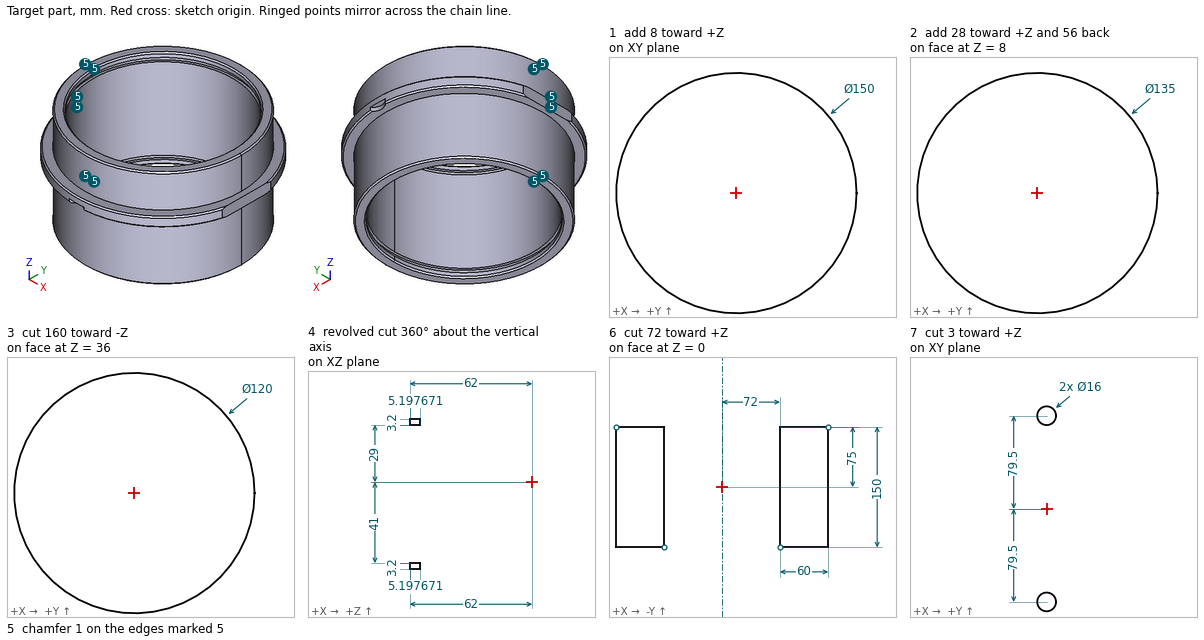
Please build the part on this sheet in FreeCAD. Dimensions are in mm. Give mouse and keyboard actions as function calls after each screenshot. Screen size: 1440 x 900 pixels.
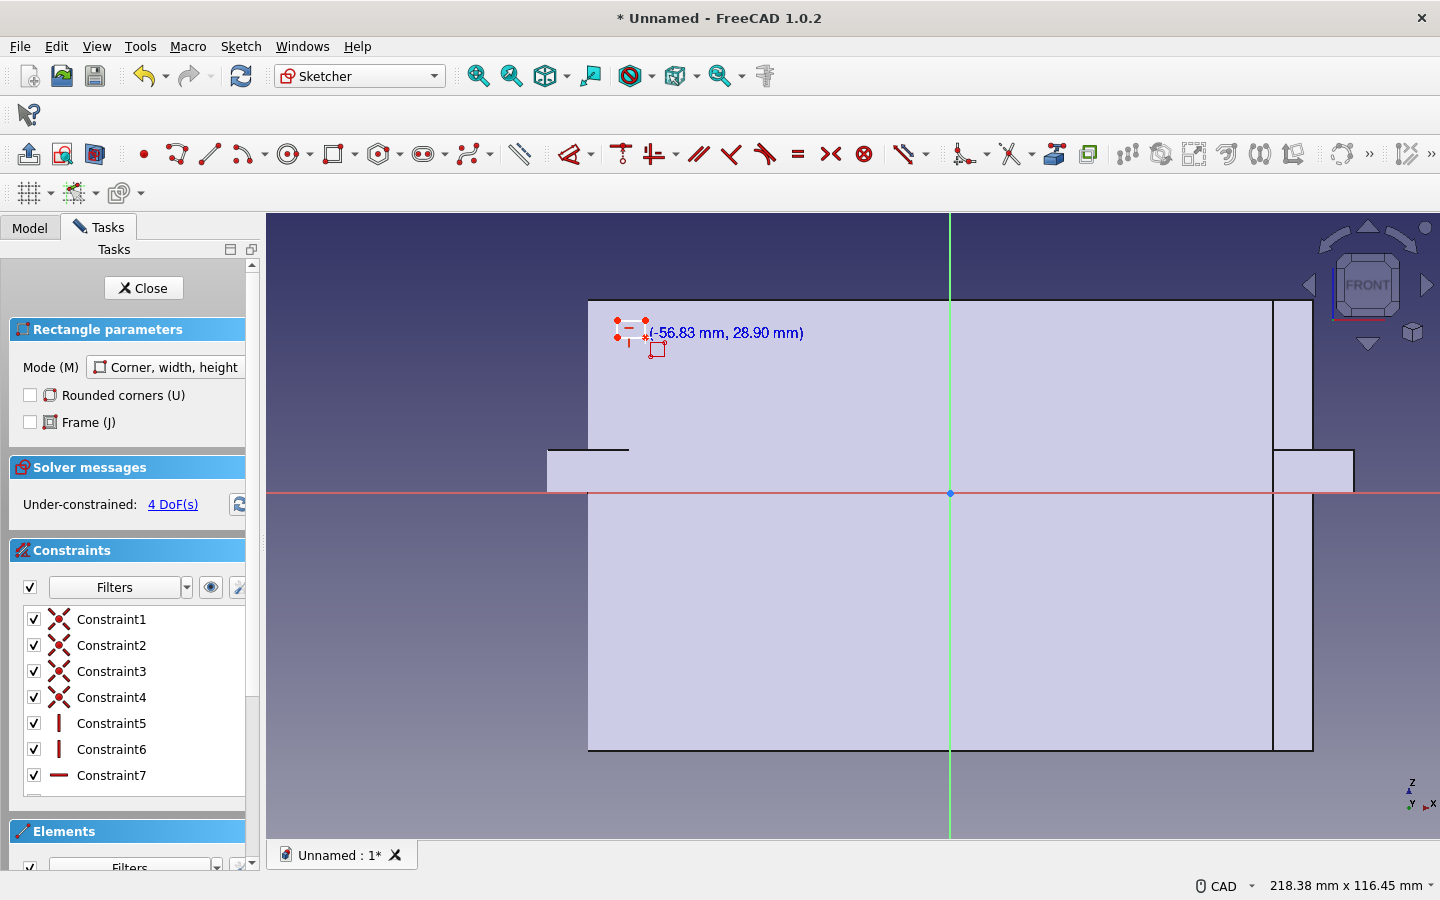
click(617, 714)
click(645, 731)
key(Escape)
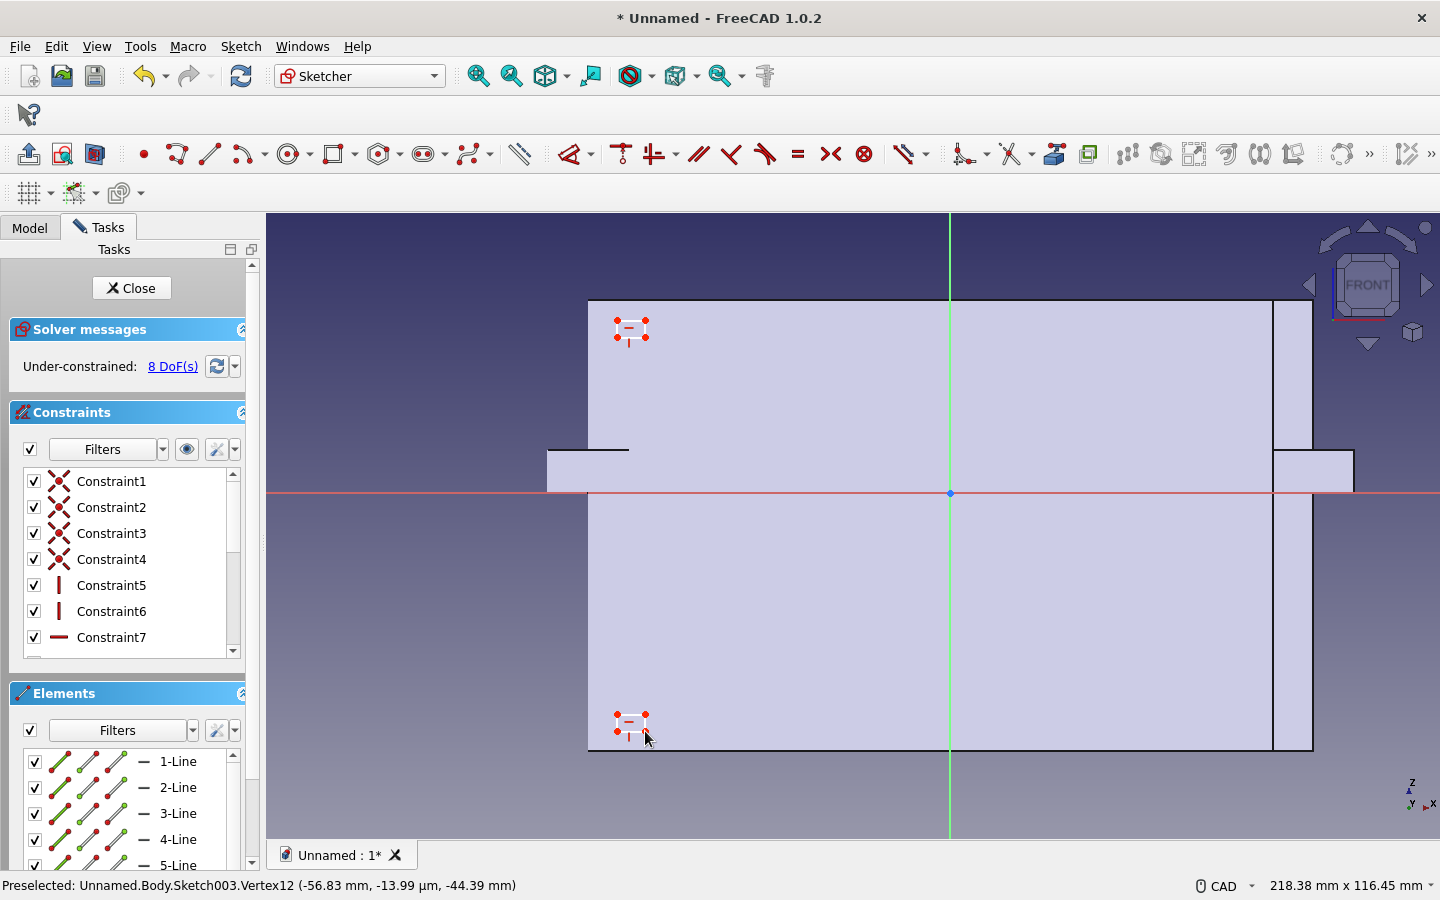
key(d)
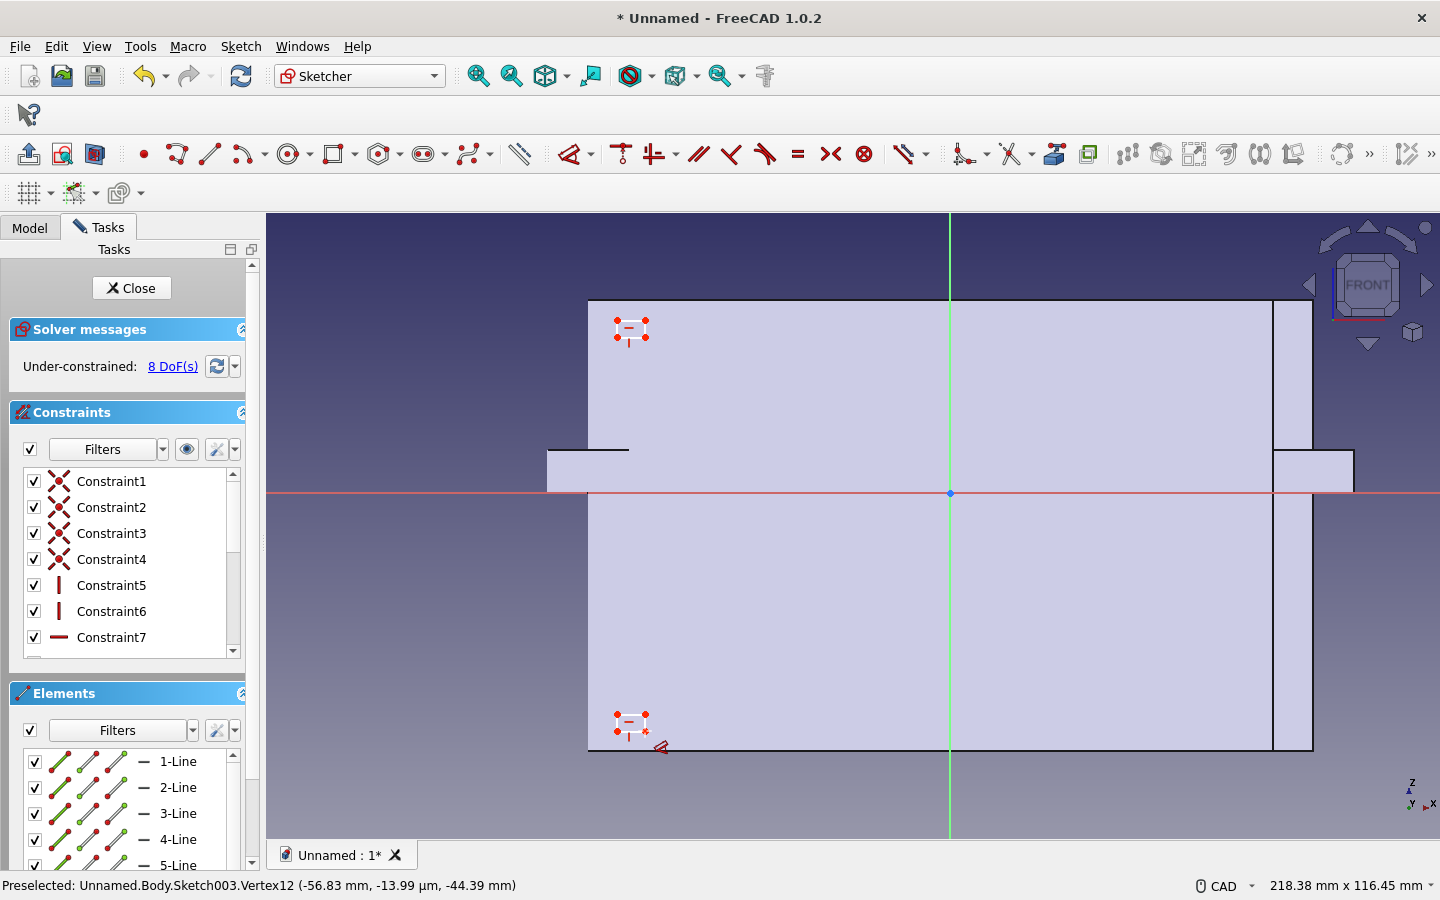
scroll(617, 329, up, 5)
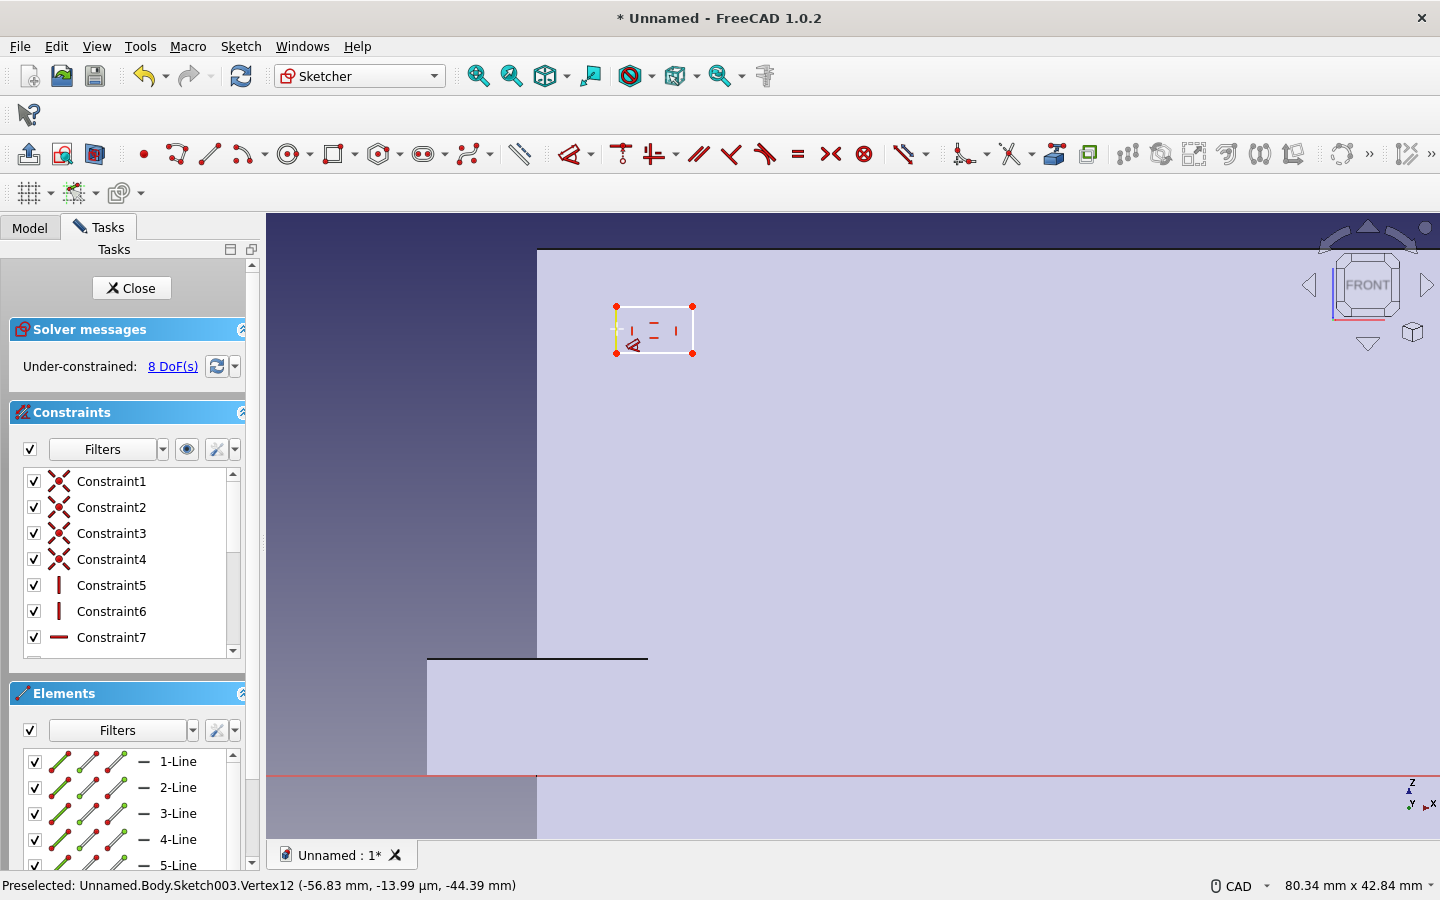
click(616, 330)
click(582, 330)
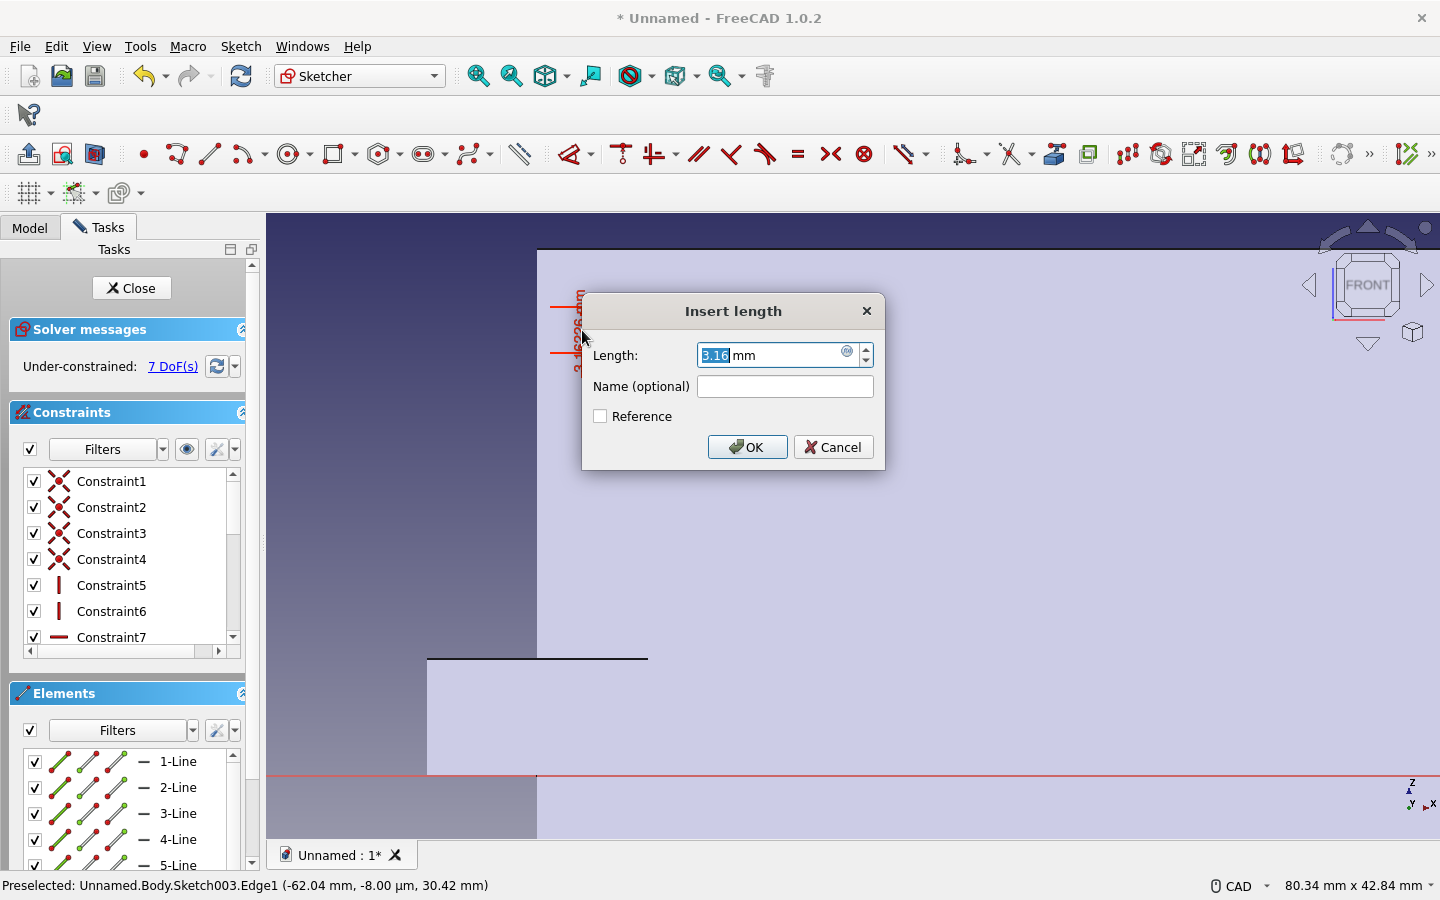
text(3.2)
key(Return)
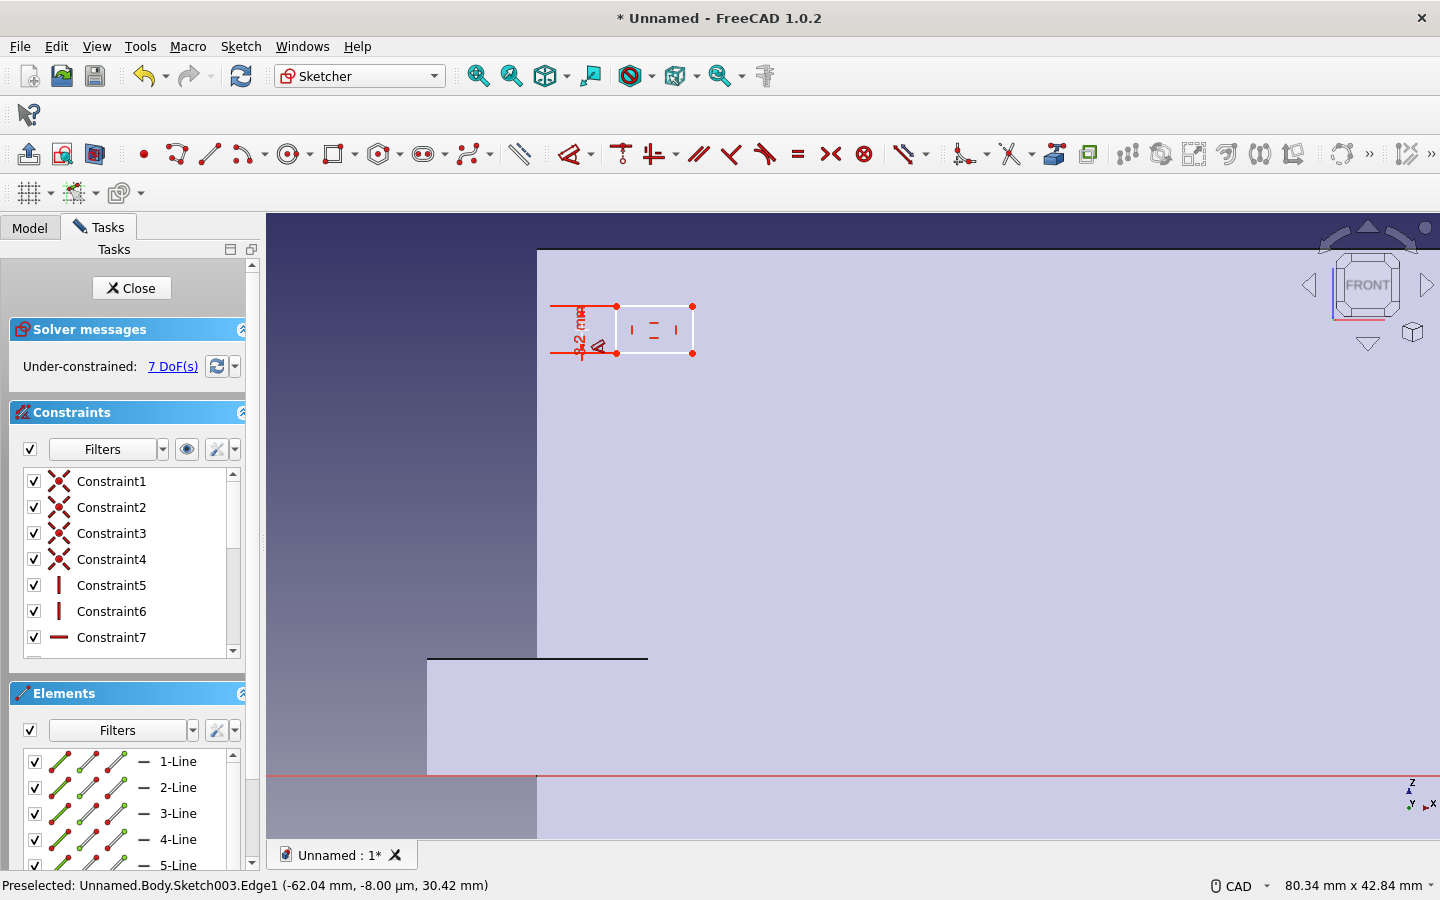
scroll(618, 330, down, 5)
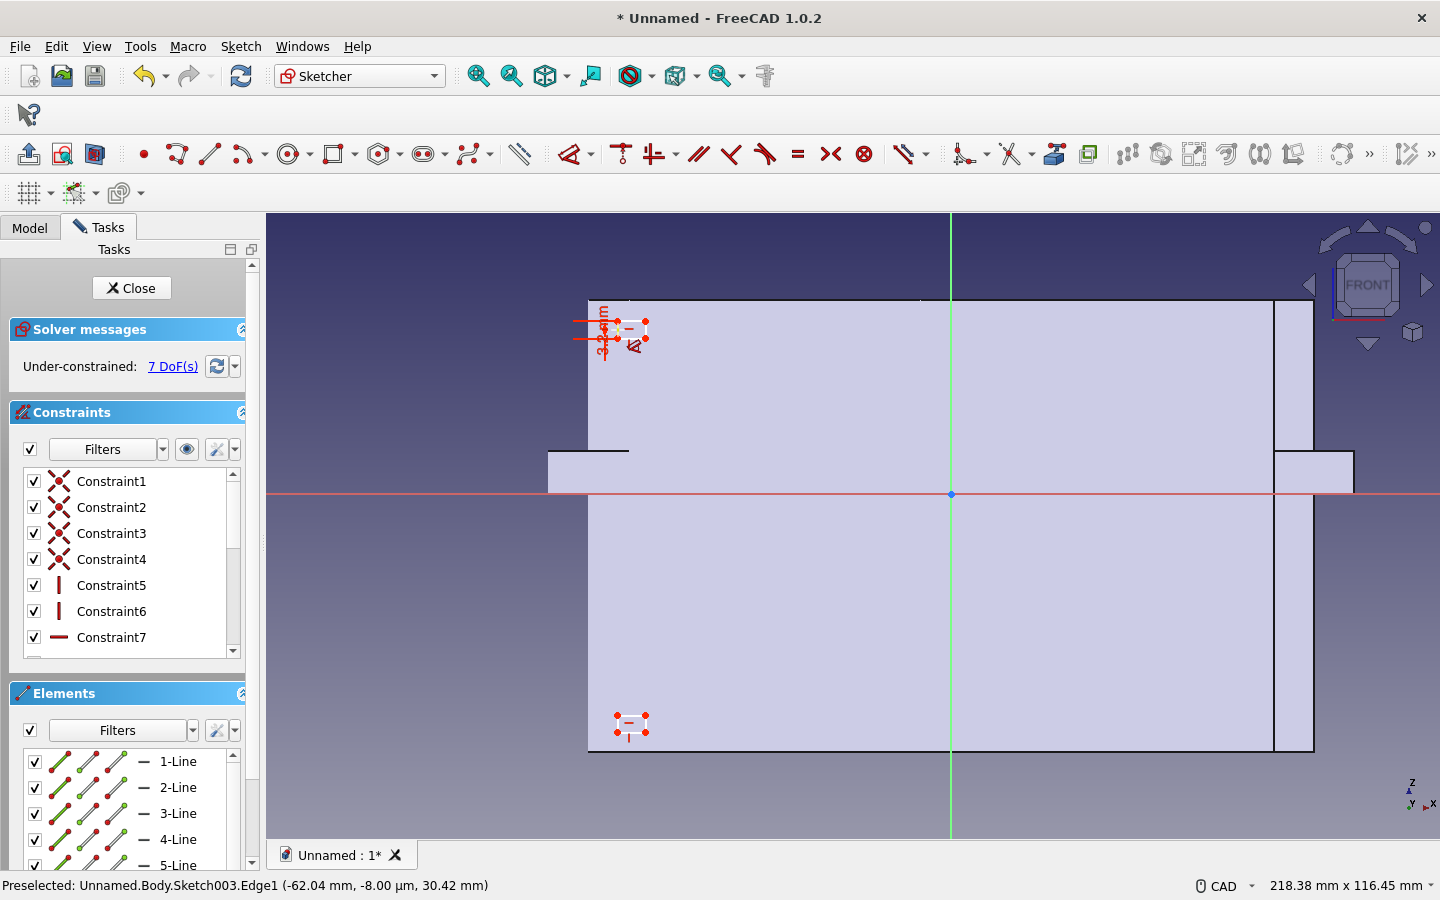
scroll(618, 721, up, 5)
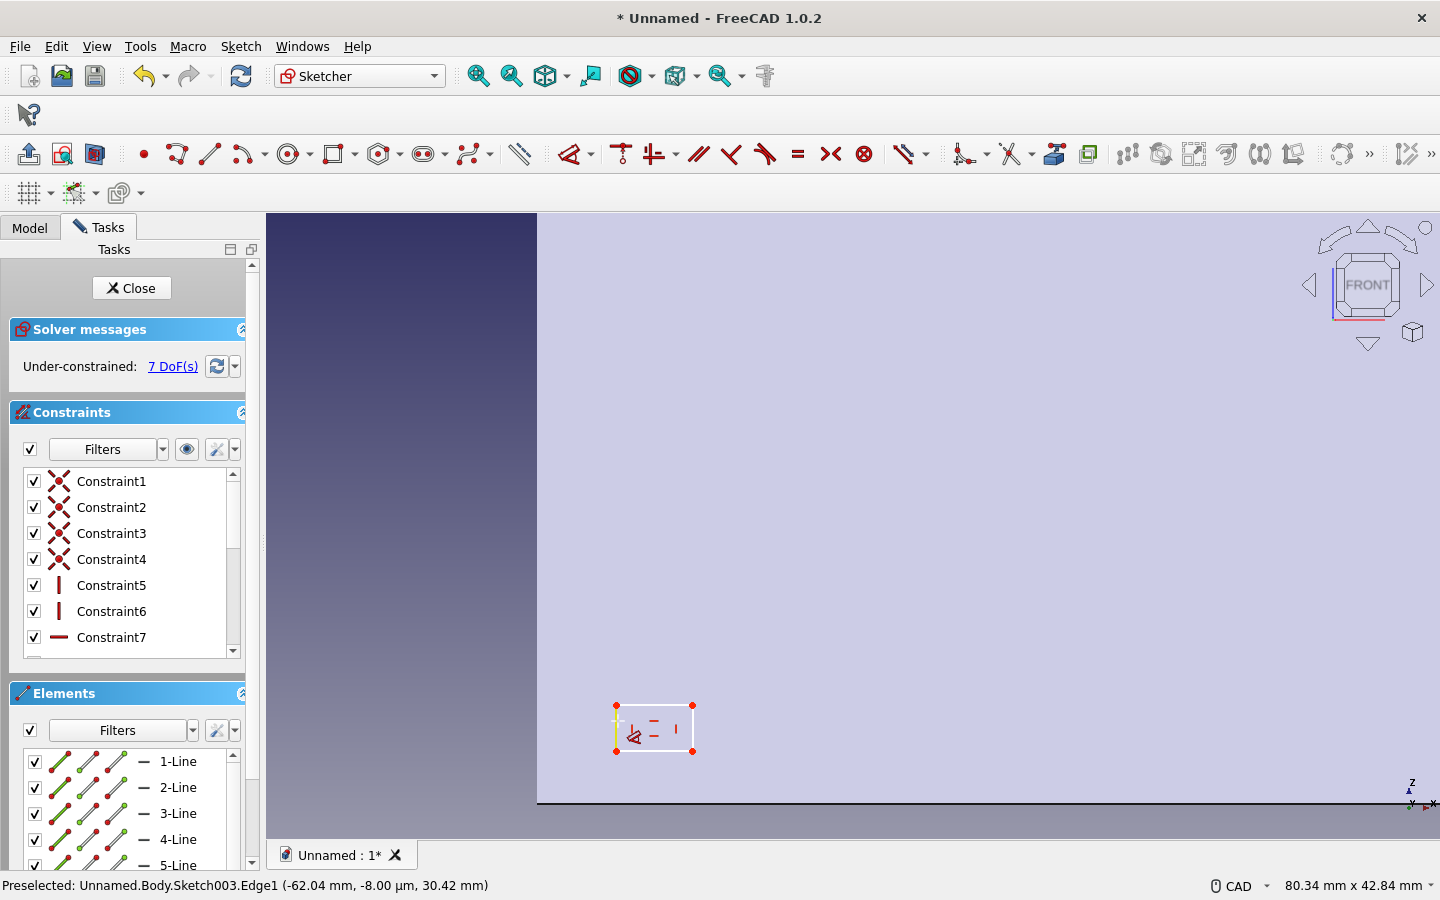
click(616, 719)
click(582, 728)